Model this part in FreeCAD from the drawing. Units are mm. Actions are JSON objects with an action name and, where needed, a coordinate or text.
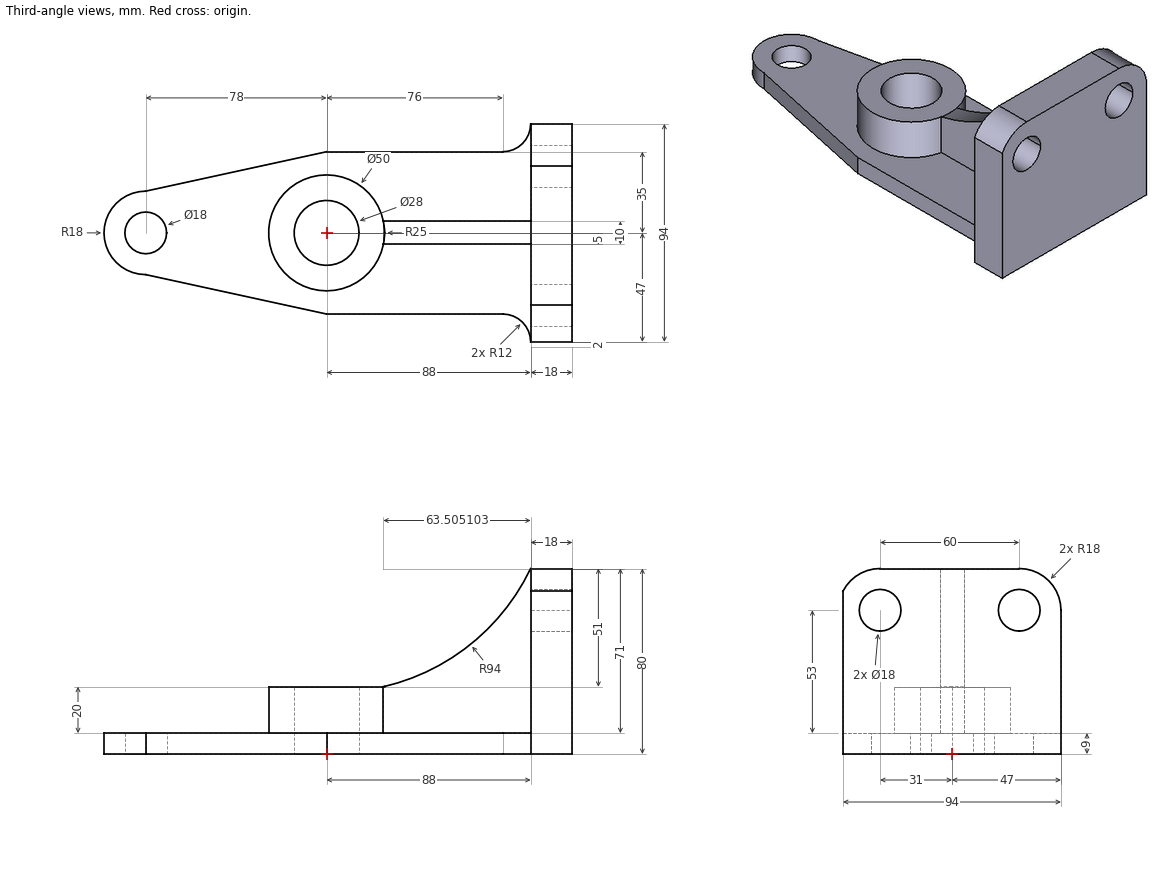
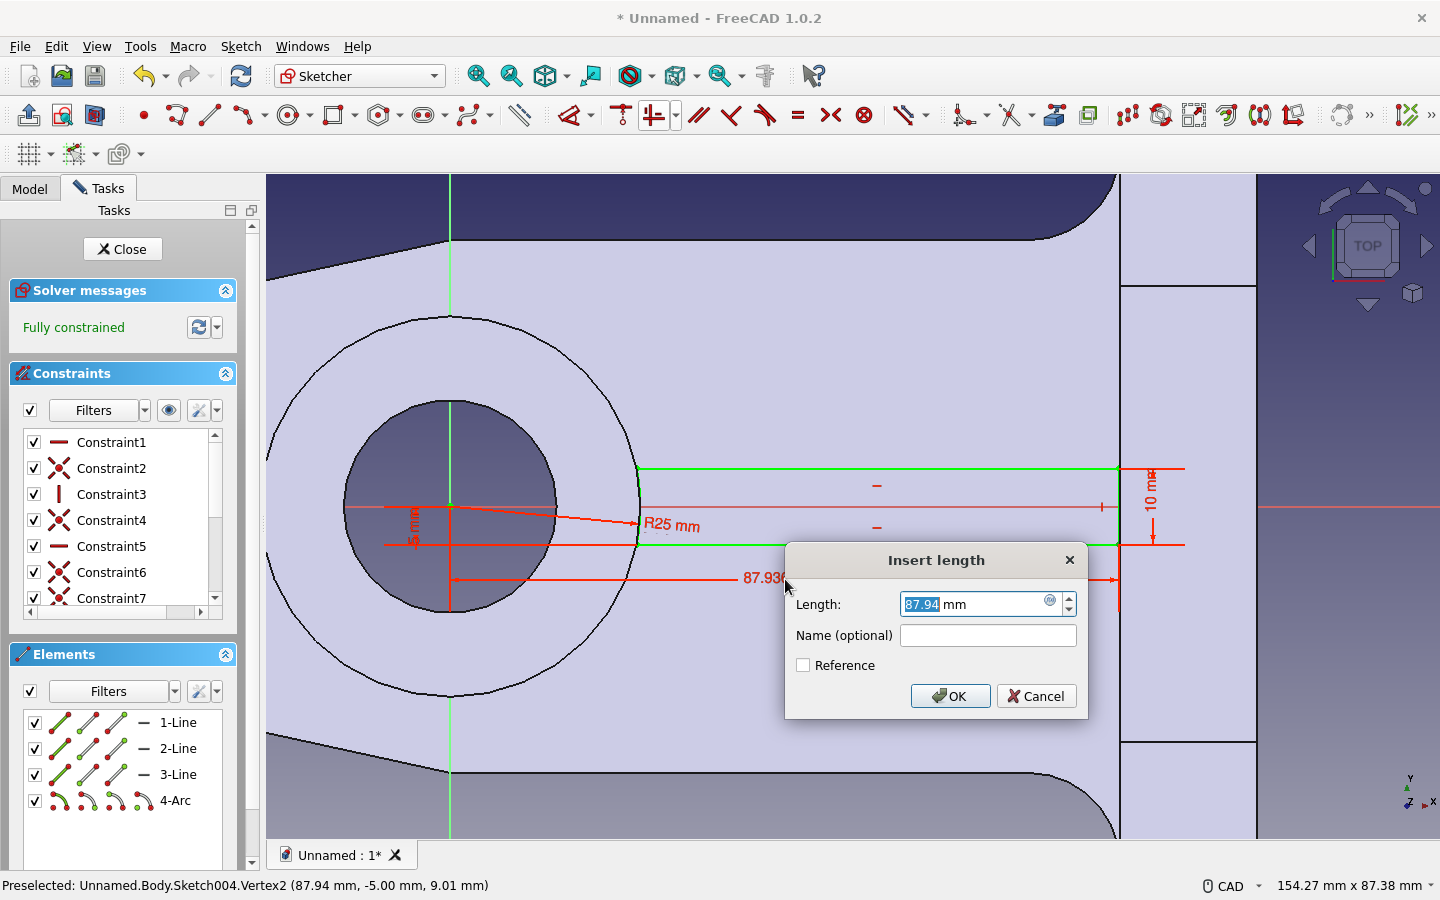
{"action": "type", "text": "88"}
{"action": "key", "text": "Return"}
{"action": "key", "text": "Escape"}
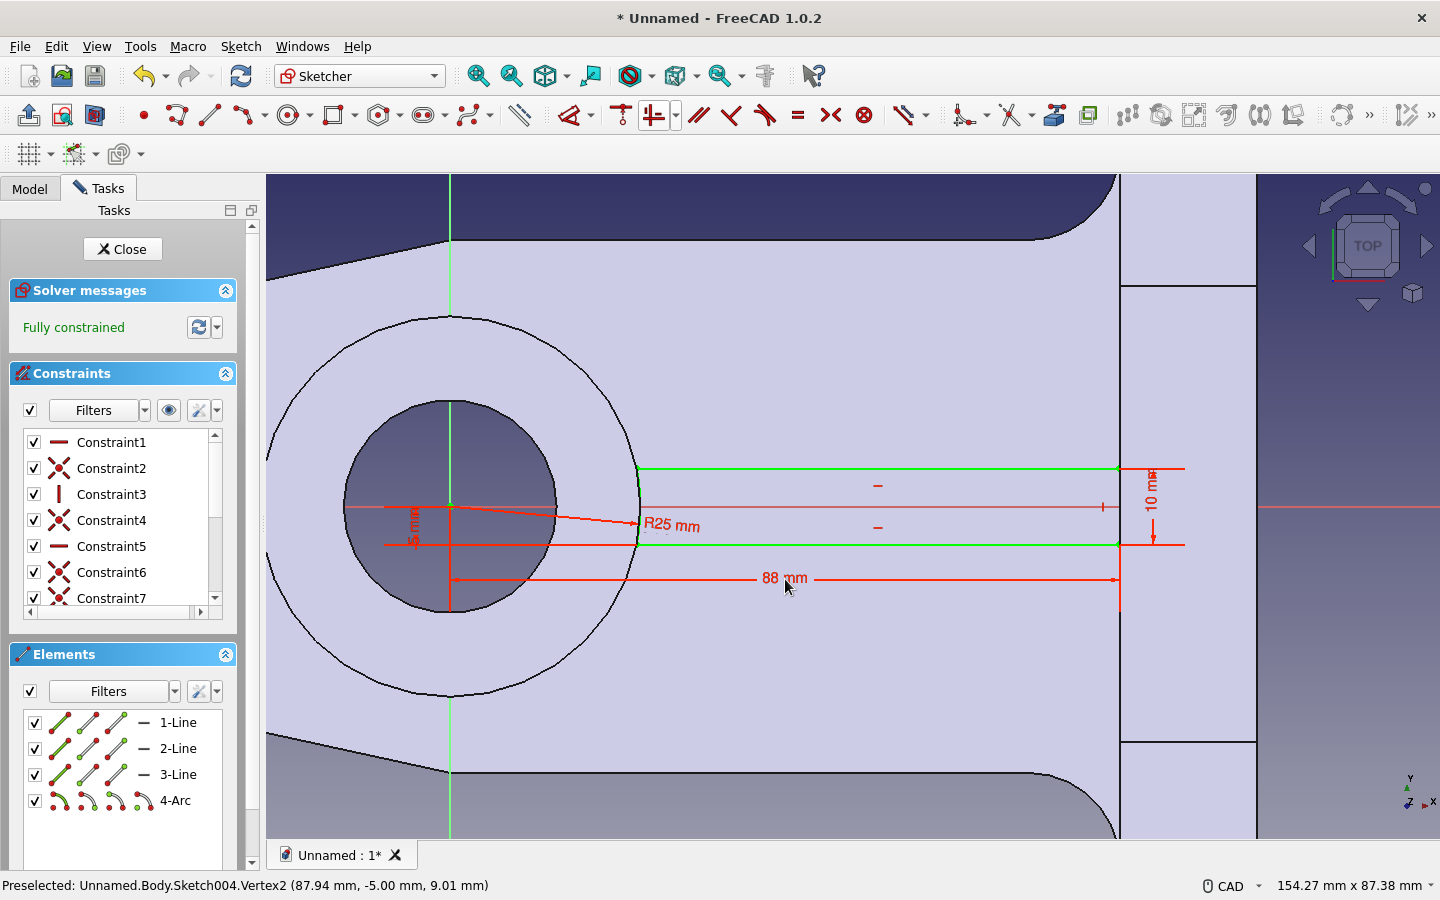
{"action": "left_click", "coordinate": [123, 249]}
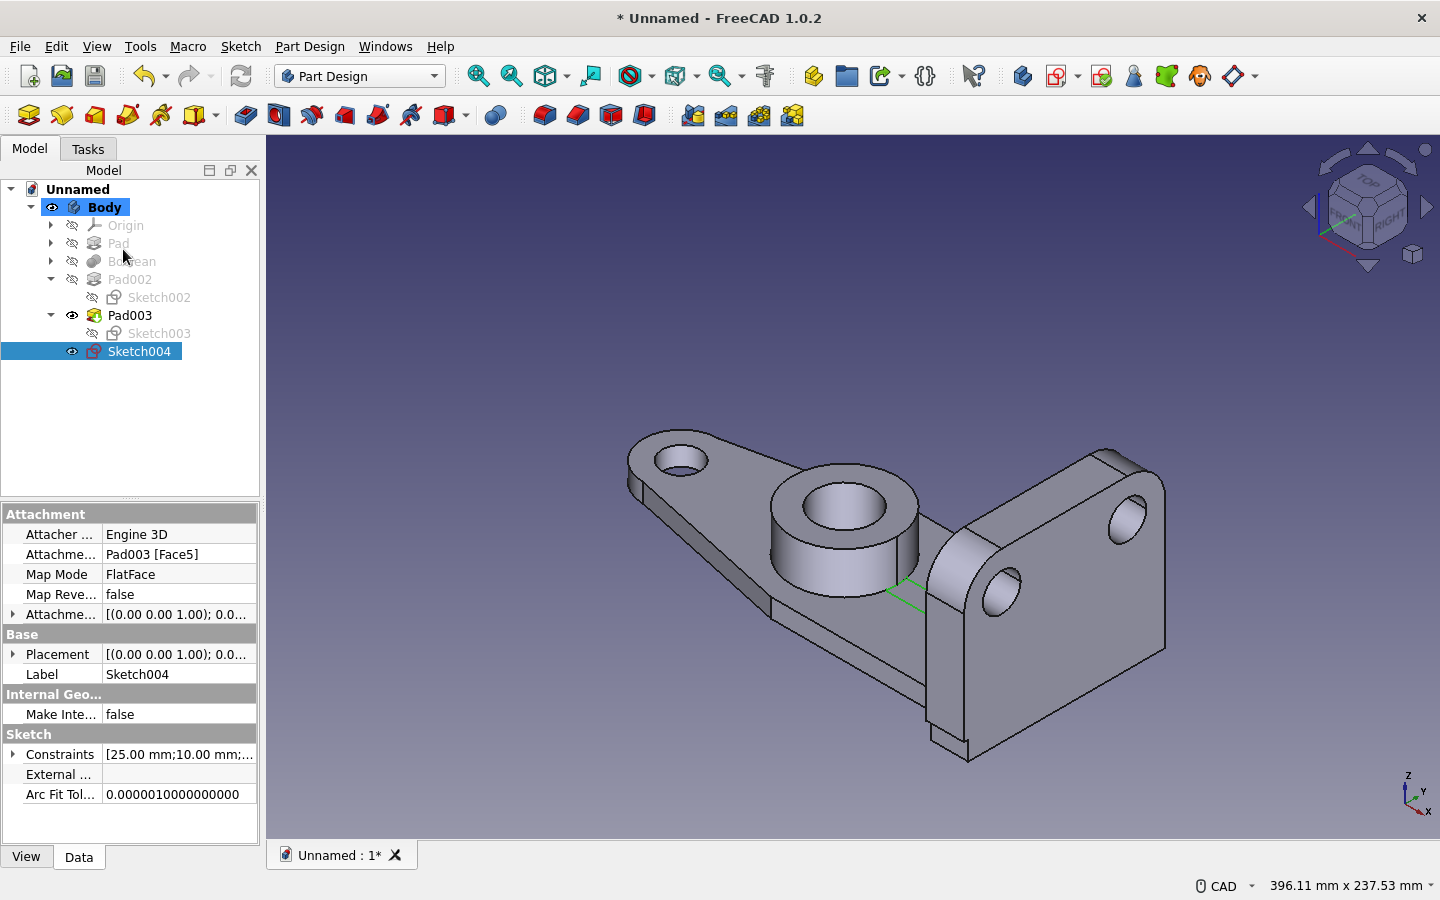
{"action": "left_click", "coordinate": [29, 116]}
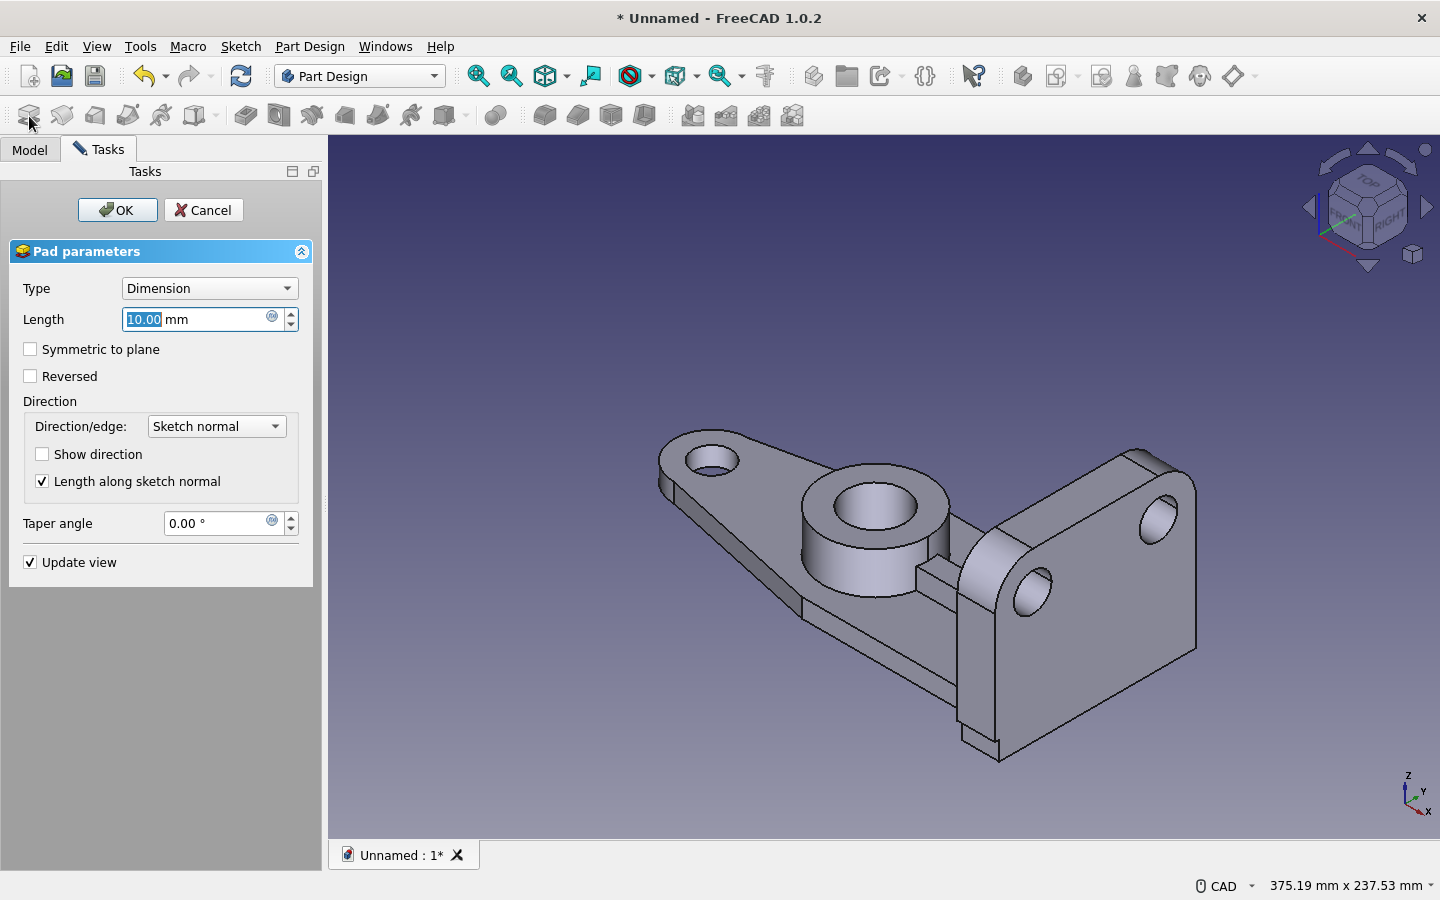
{"action": "type", "text": "71"}
{"action": "key", "text": "Tab"}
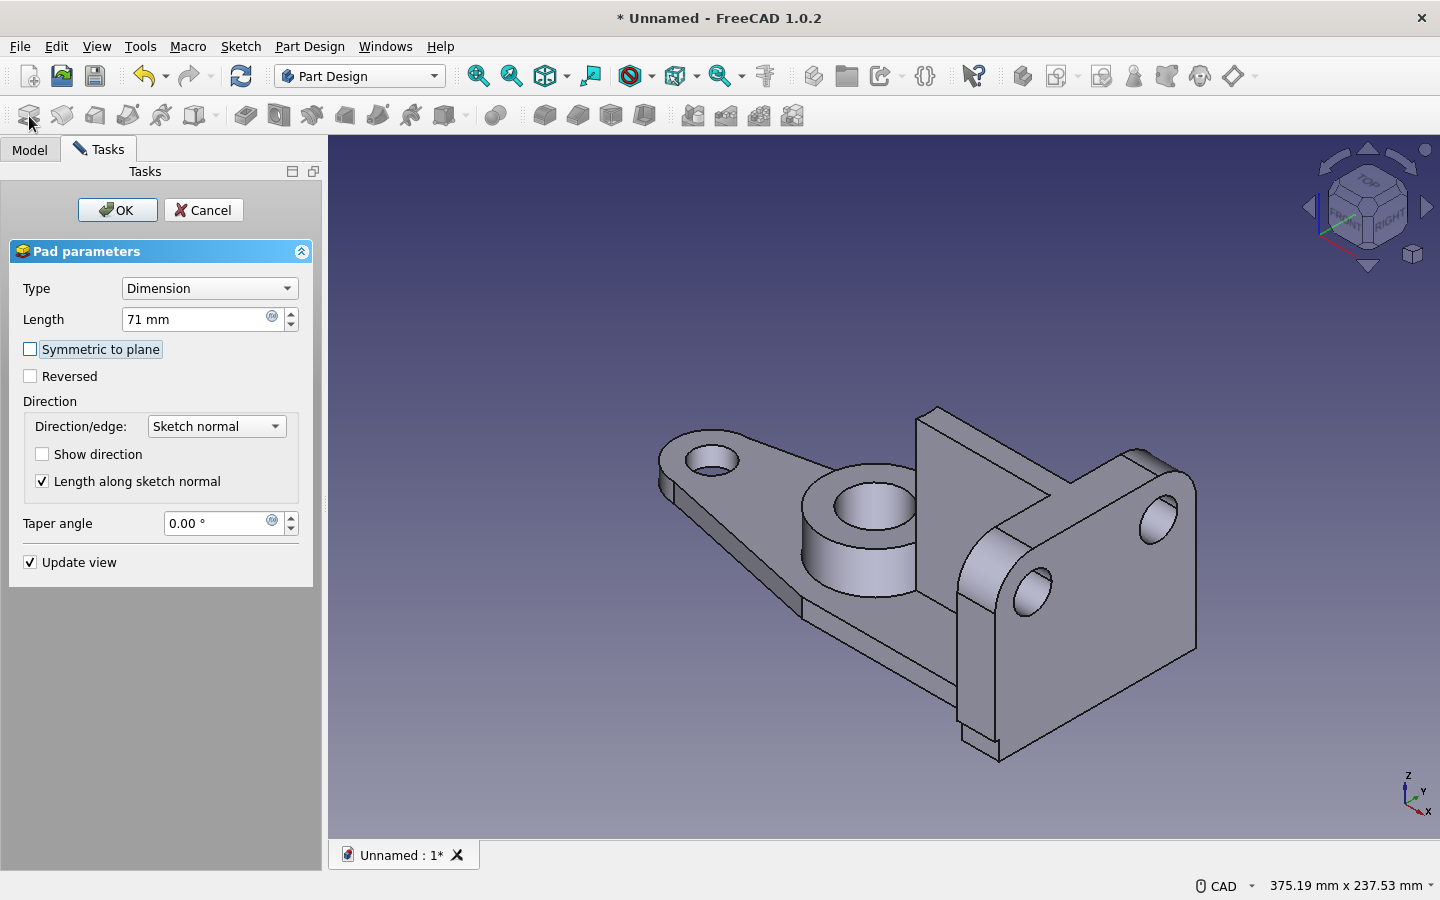
{"action": "left_click", "coordinate": [118, 210]}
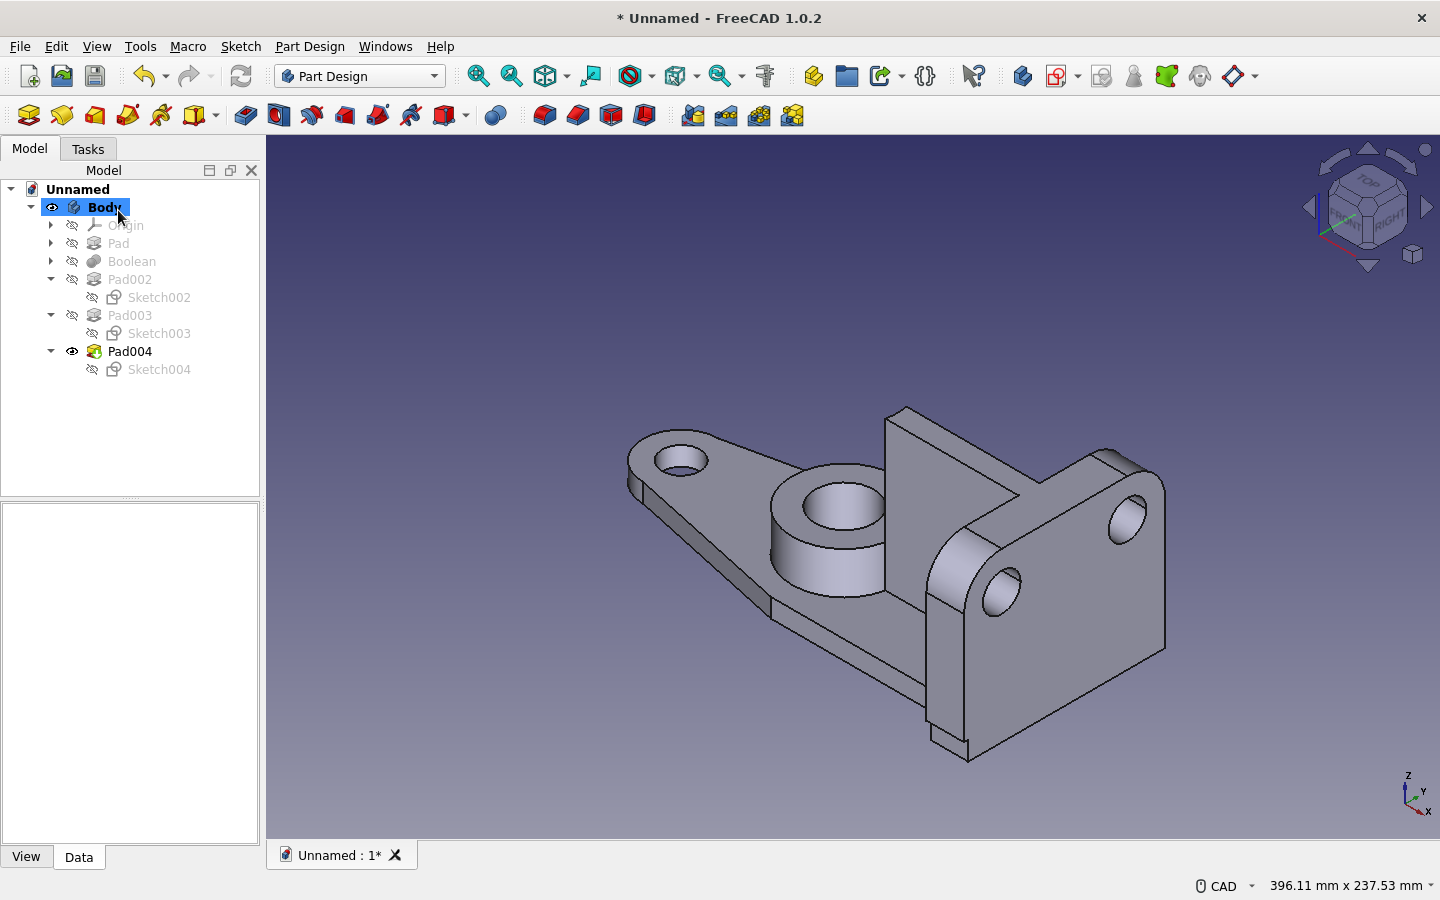
{"action": "left_click", "coordinate": [952, 517]}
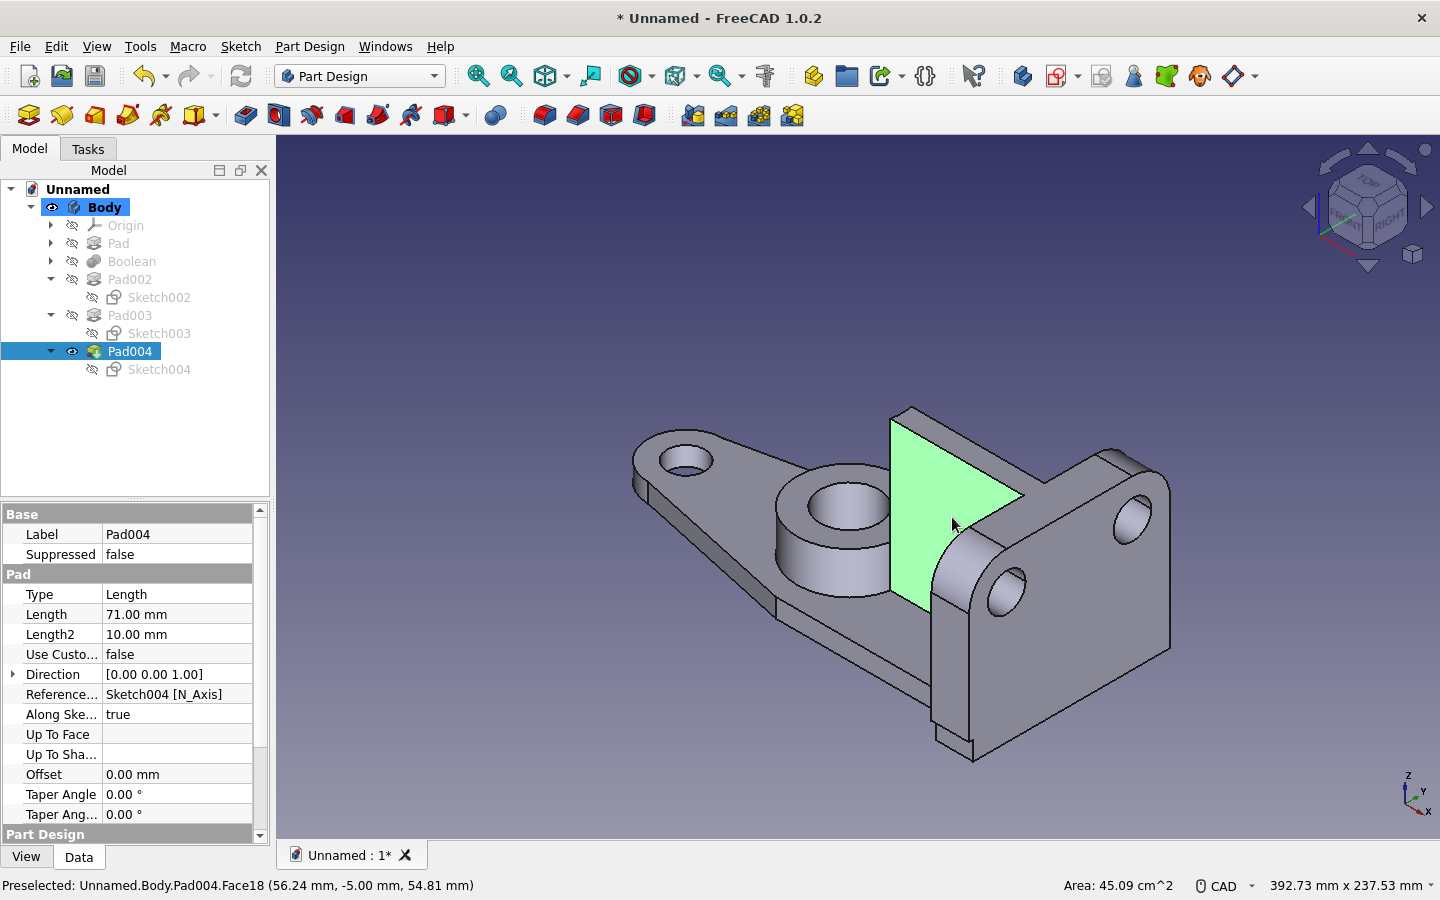
{"action": "left_click", "coordinate": [1056, 76]}